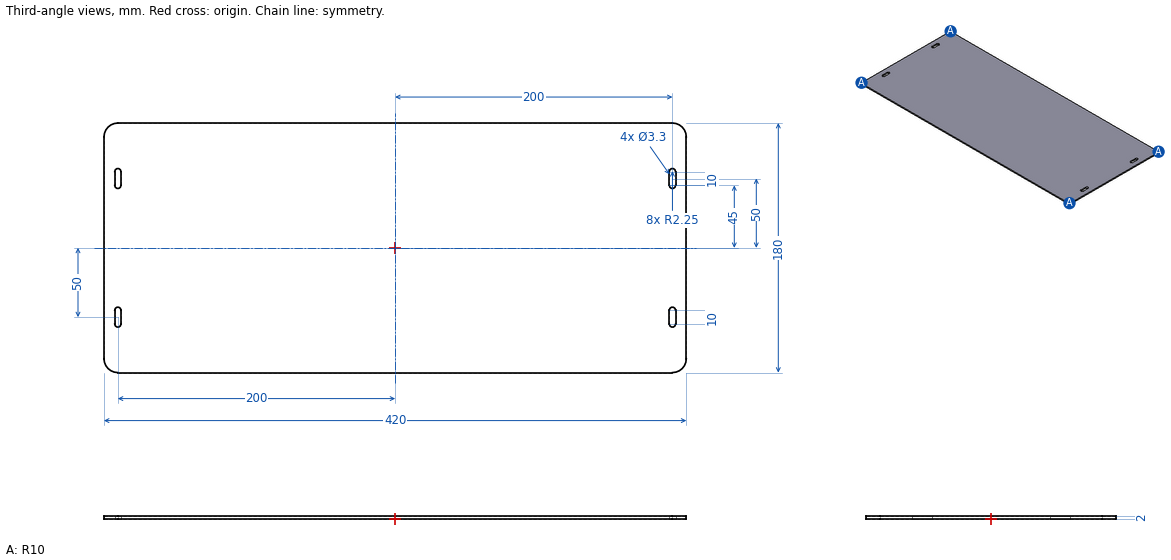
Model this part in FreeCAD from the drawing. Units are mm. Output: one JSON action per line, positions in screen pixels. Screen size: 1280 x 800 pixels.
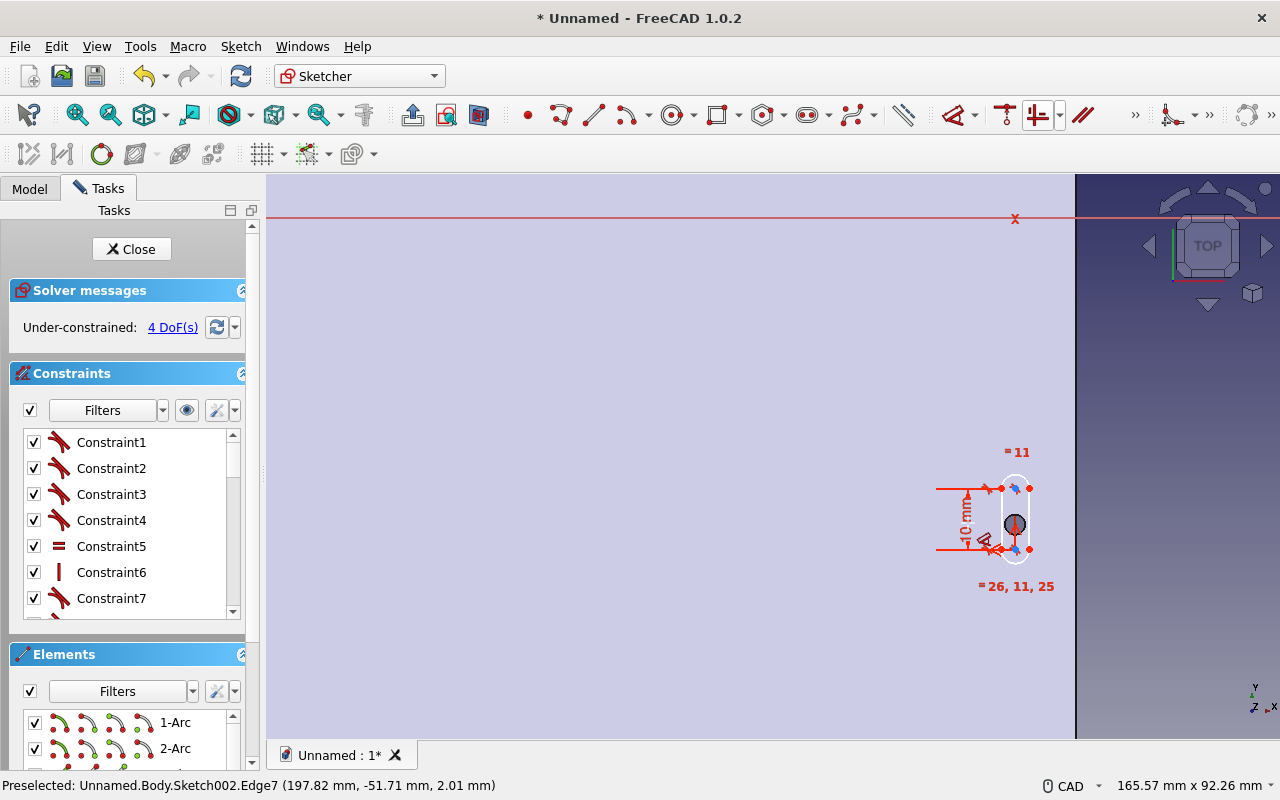
{"action": "scroll", "coordinate": [1004, 534], "scroll_direction": "down", "scroll_amount": 7}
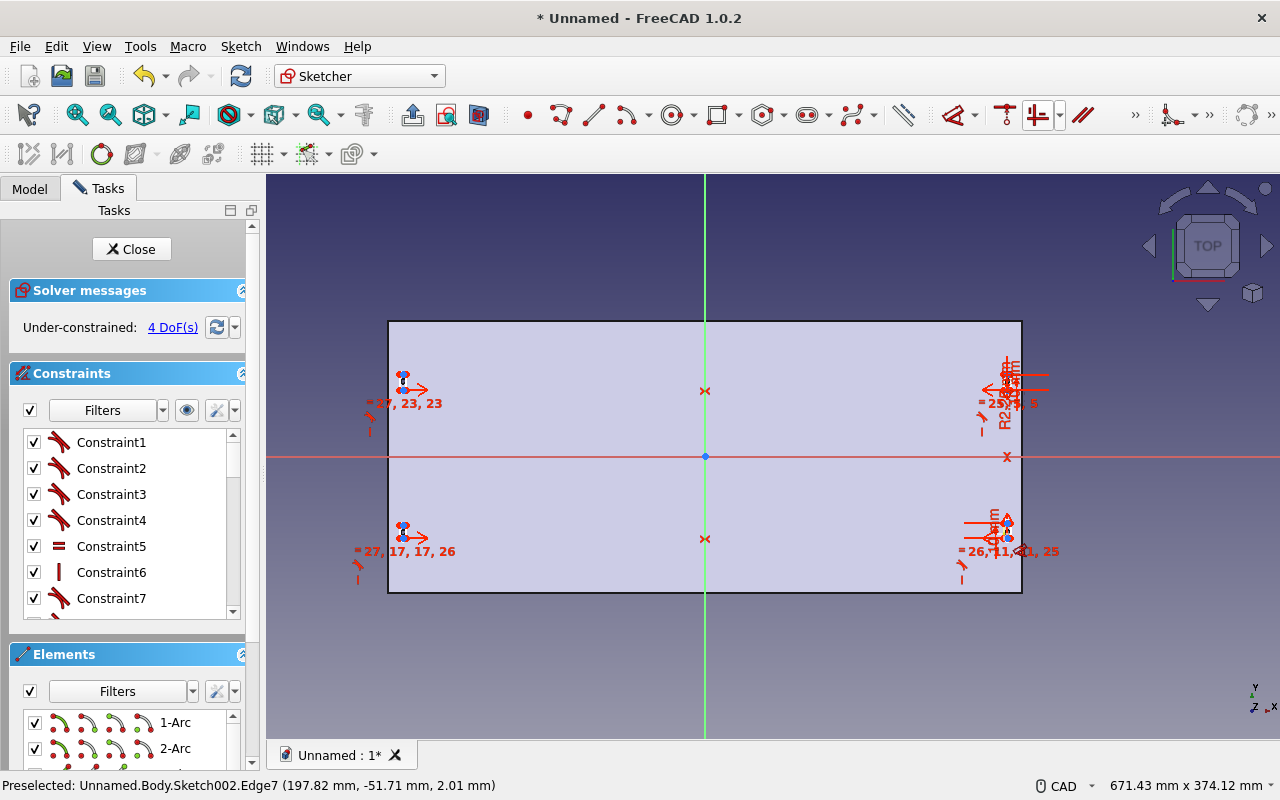
{"action": "scroll", "coordinate": [400, 535], "scroll_direction": "up", "scroll_amount": 7}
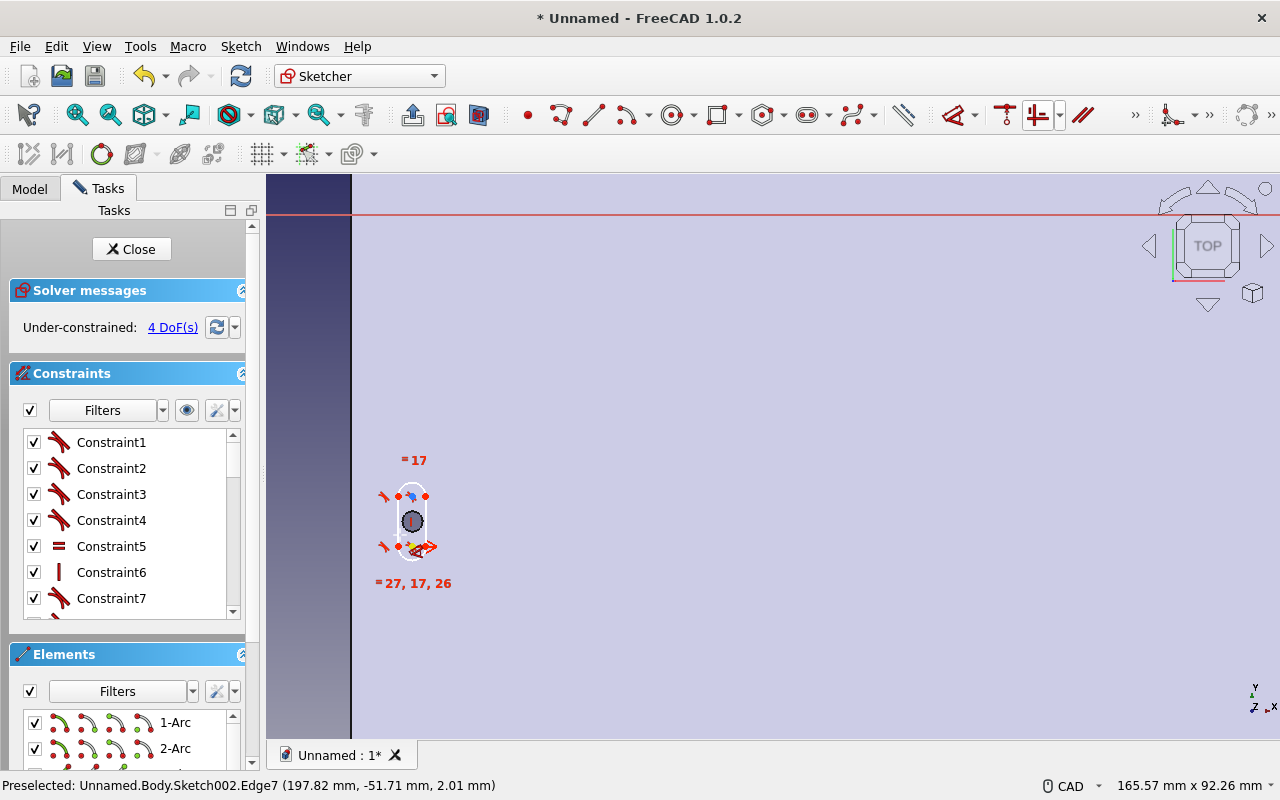
{"action": "left_click", "coordinate": [398, 532]}
{"action": "left_click", "coordinate": [364, 522]}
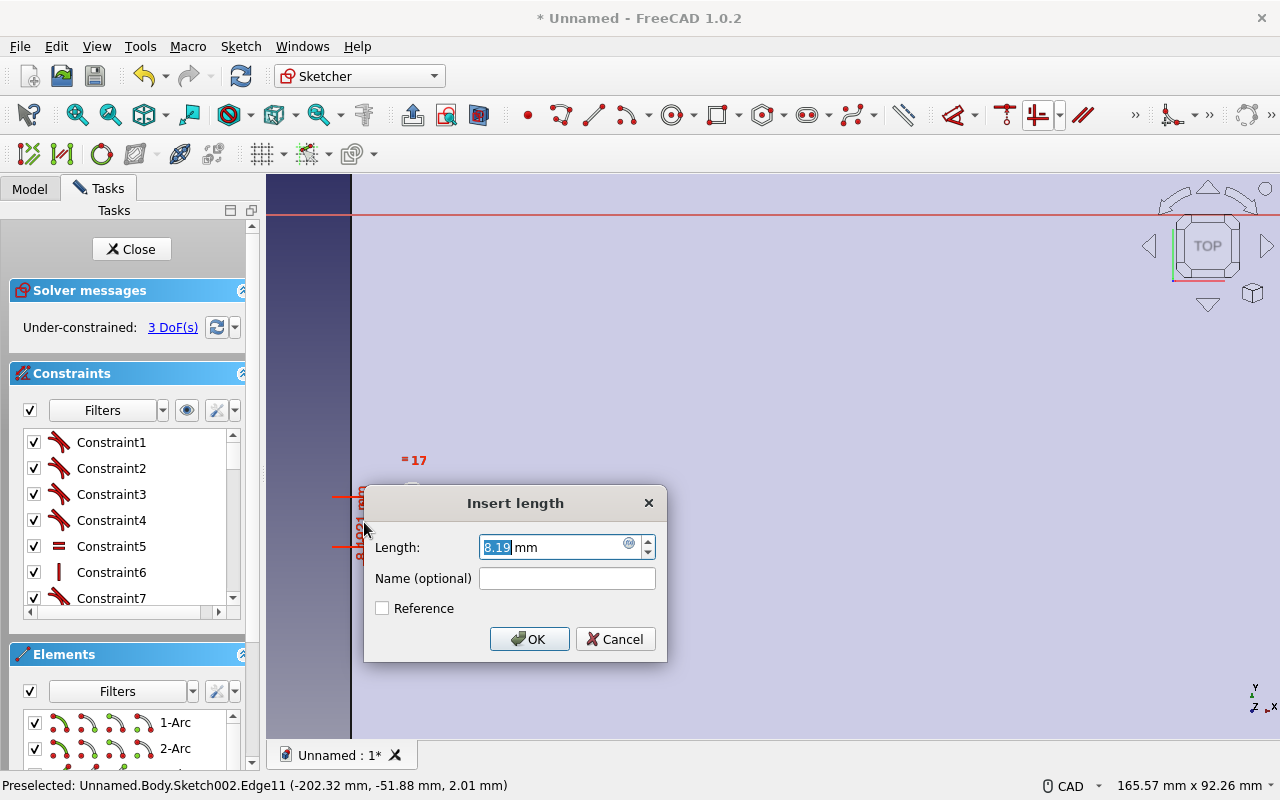
{"action": "type", "text": "10"}
{"action": "key", "text": "Return"}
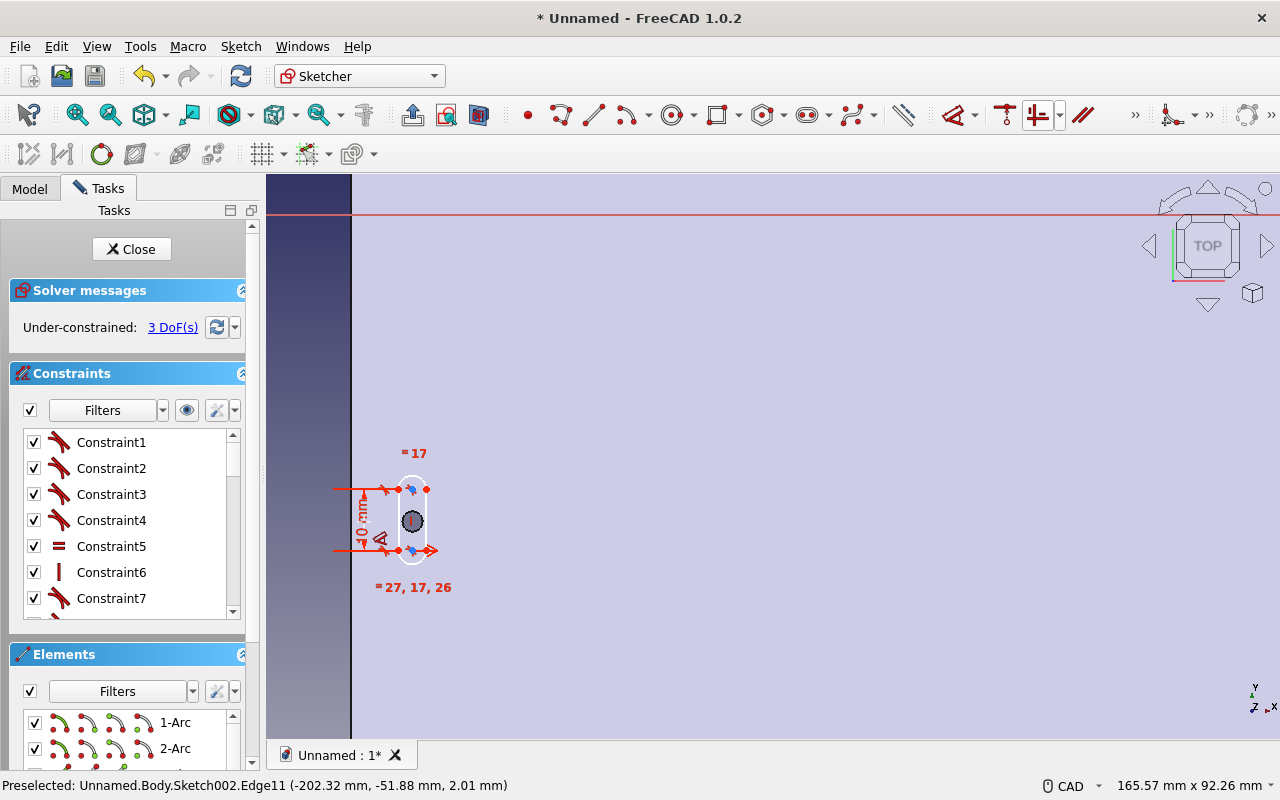
{"action": "scroll", "coordinate": [399, 535], "scroll_direction": "down", "scroll_amount": 7}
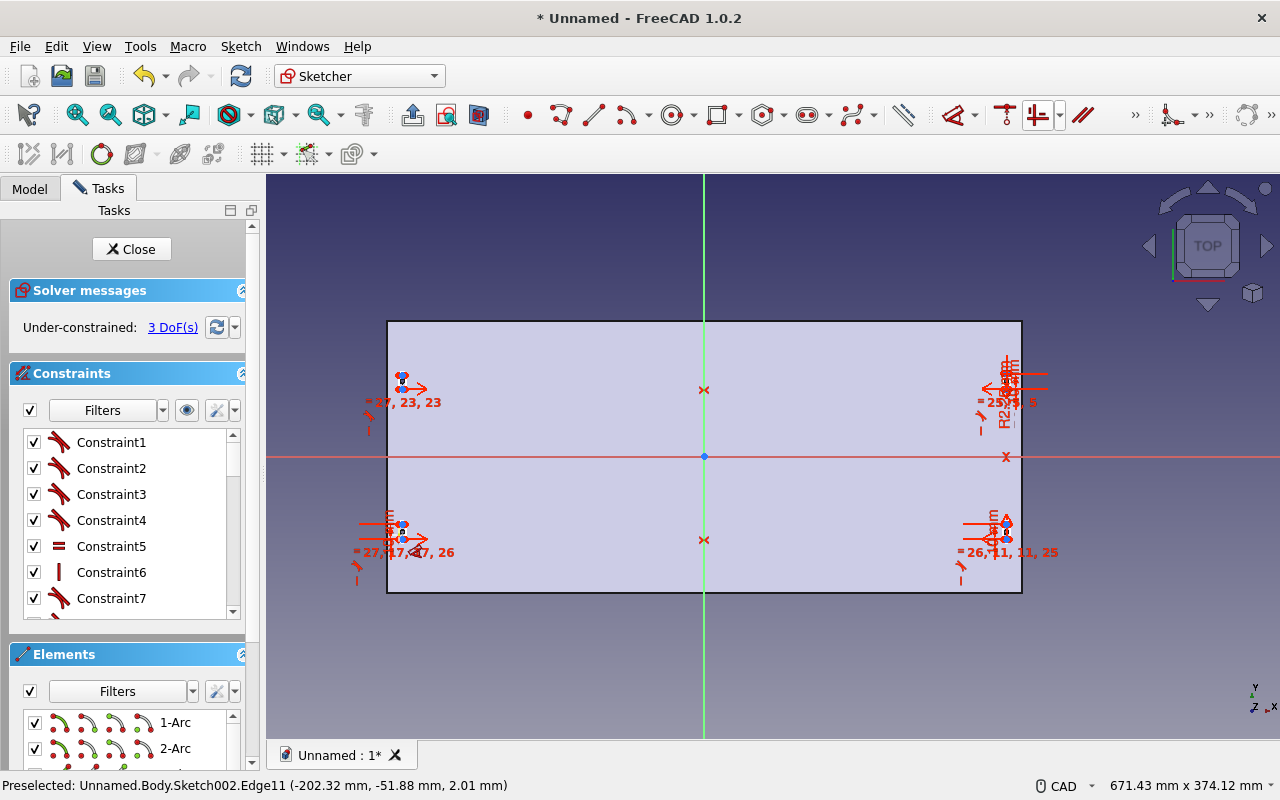
{"action": "scroll", "coordinate": [399, 385], "scroll_direction": "up", "scroll_amount": 6}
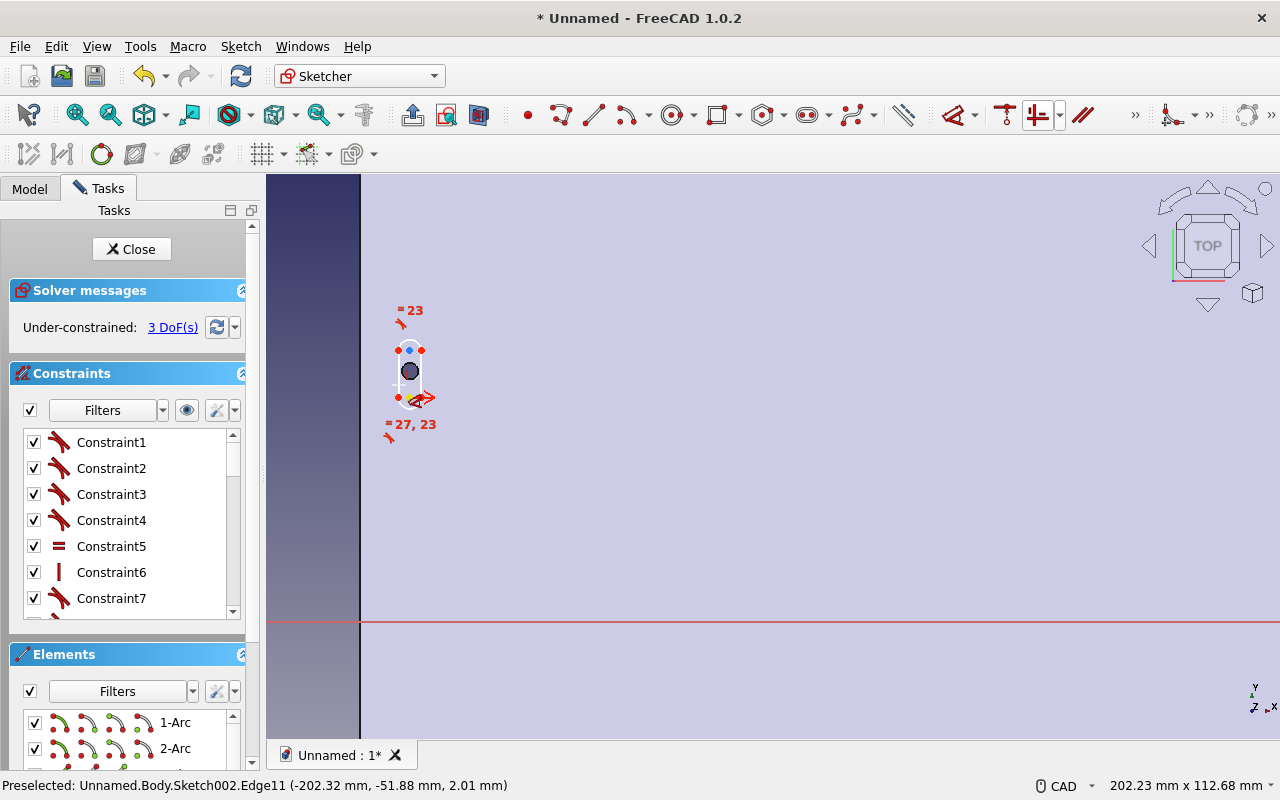
{"action": "left_click", "coordinate": [399, 384]}
{"action": "left_click", "coordinate": [365, 374]}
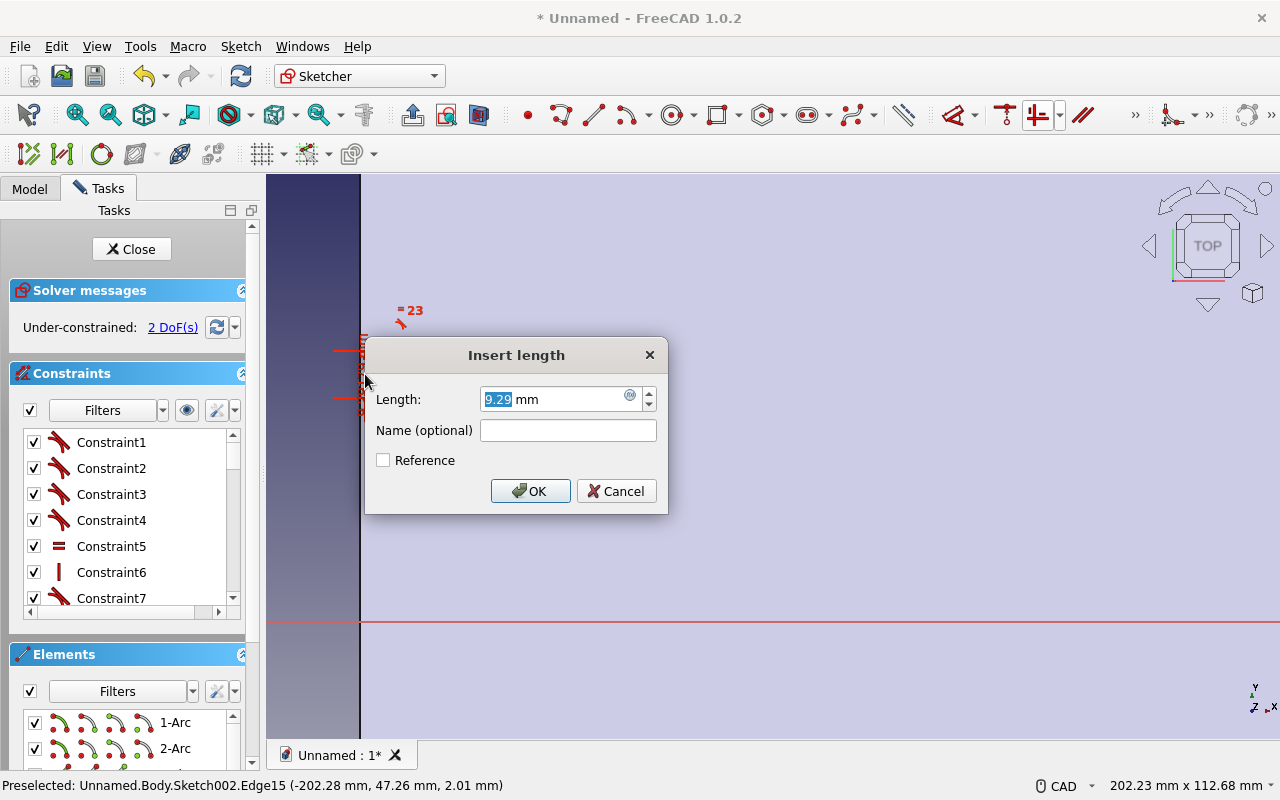
{"action": "type", "text": "10"}
{"action": "key", "text": "Return"}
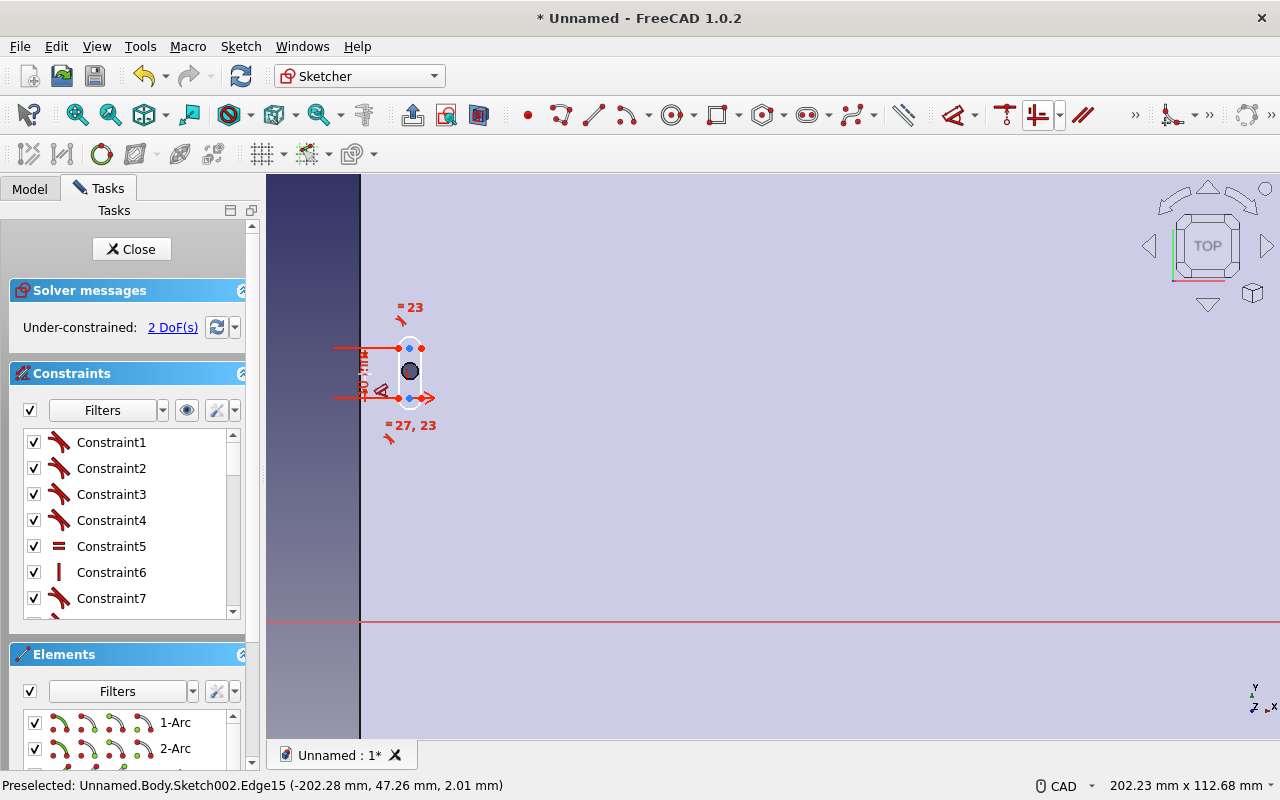
{"action": "scroll", "coordinate": [399, 385], "scroll_direction": "down", "scroll_amount": 6}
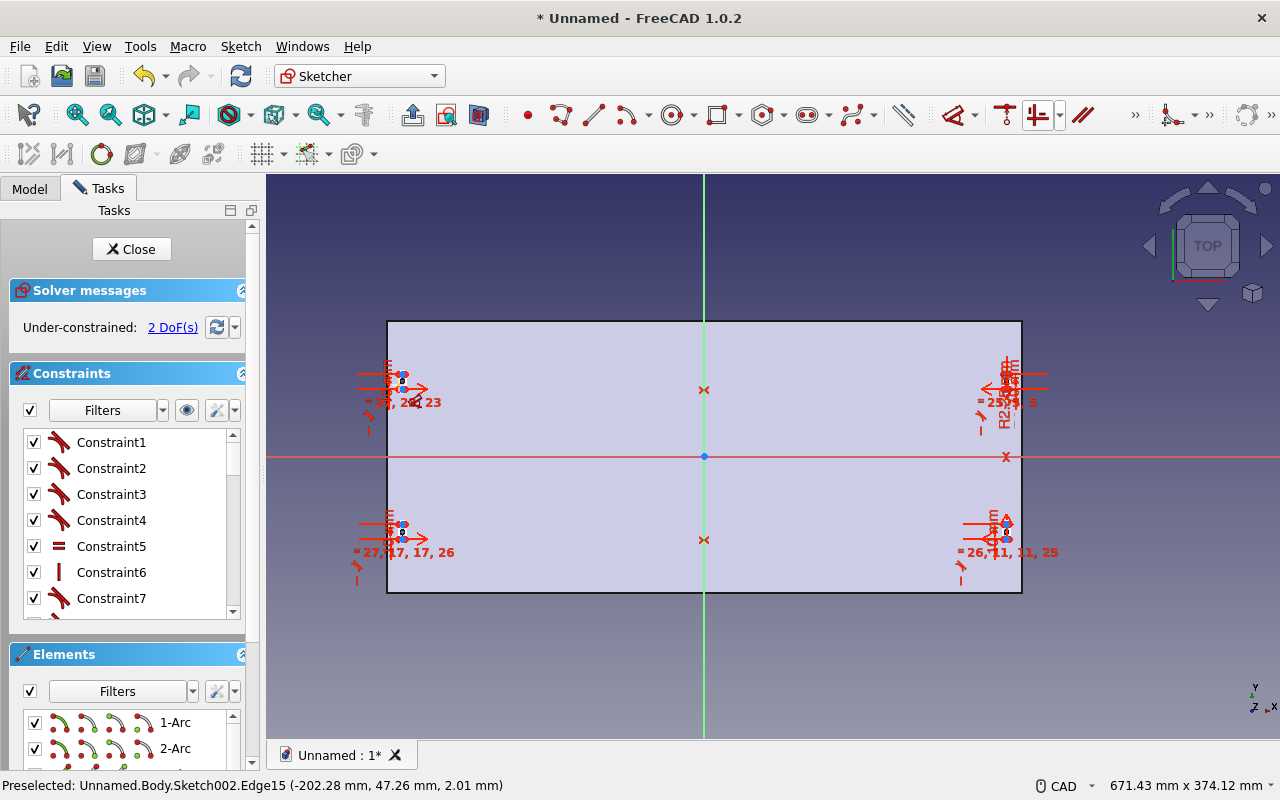
{"action": "scroll", "coordinate": [1003, 389], "scroll_direction": "up", "scroll_amount": 7}